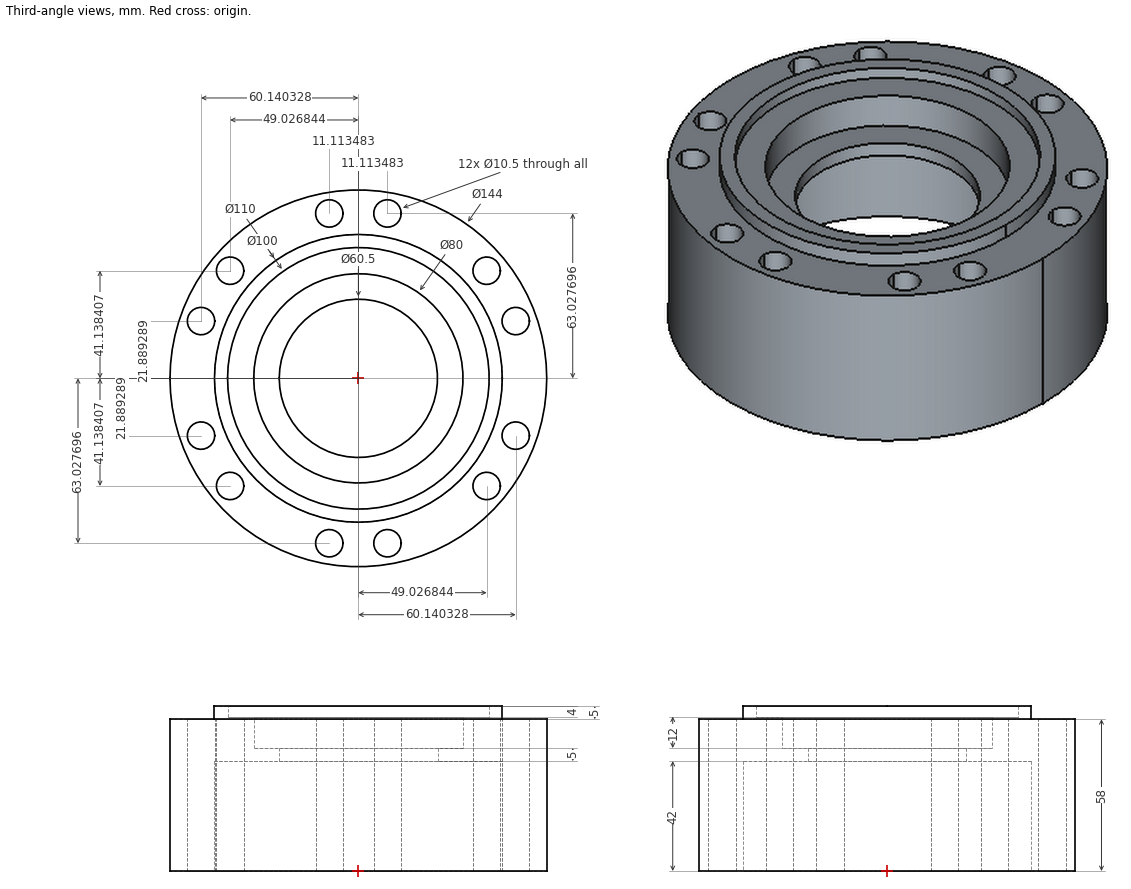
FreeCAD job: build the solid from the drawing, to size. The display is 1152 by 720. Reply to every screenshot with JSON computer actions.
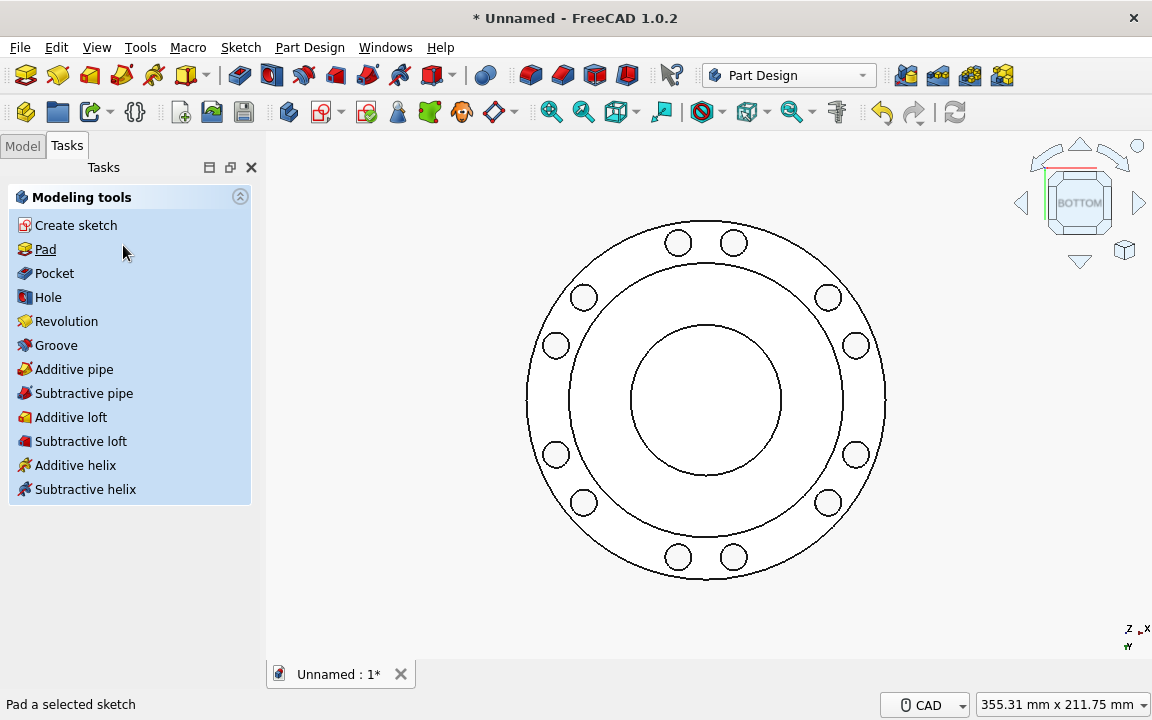
{"action": "left_click", "coordinate": [240, 76]}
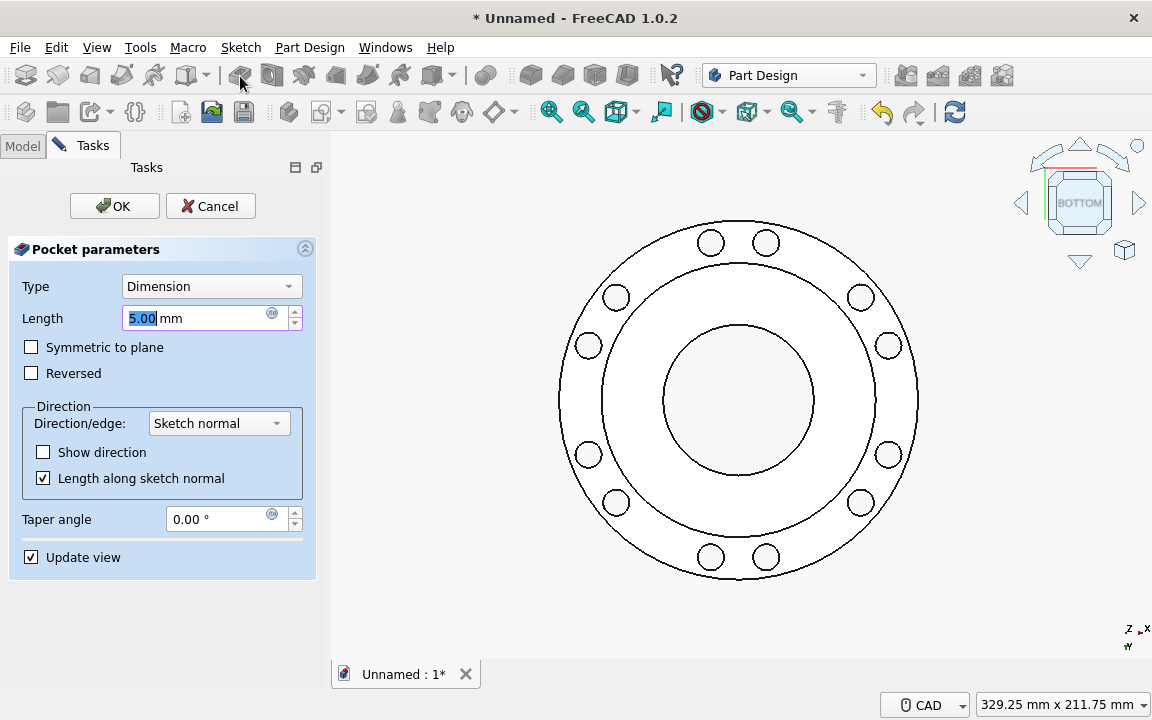
{"action": "type", "text": "4"}
{"action": "key", "text": "Tab"}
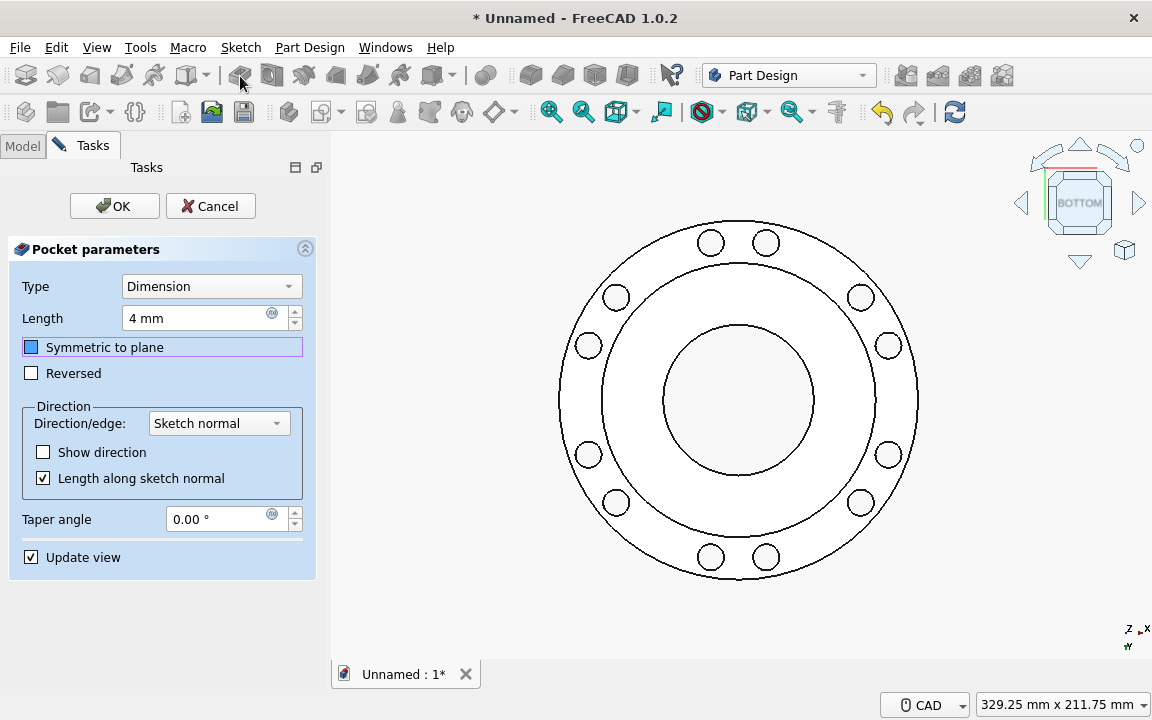
{"action": "left_click", "coordinate": [115, 206]}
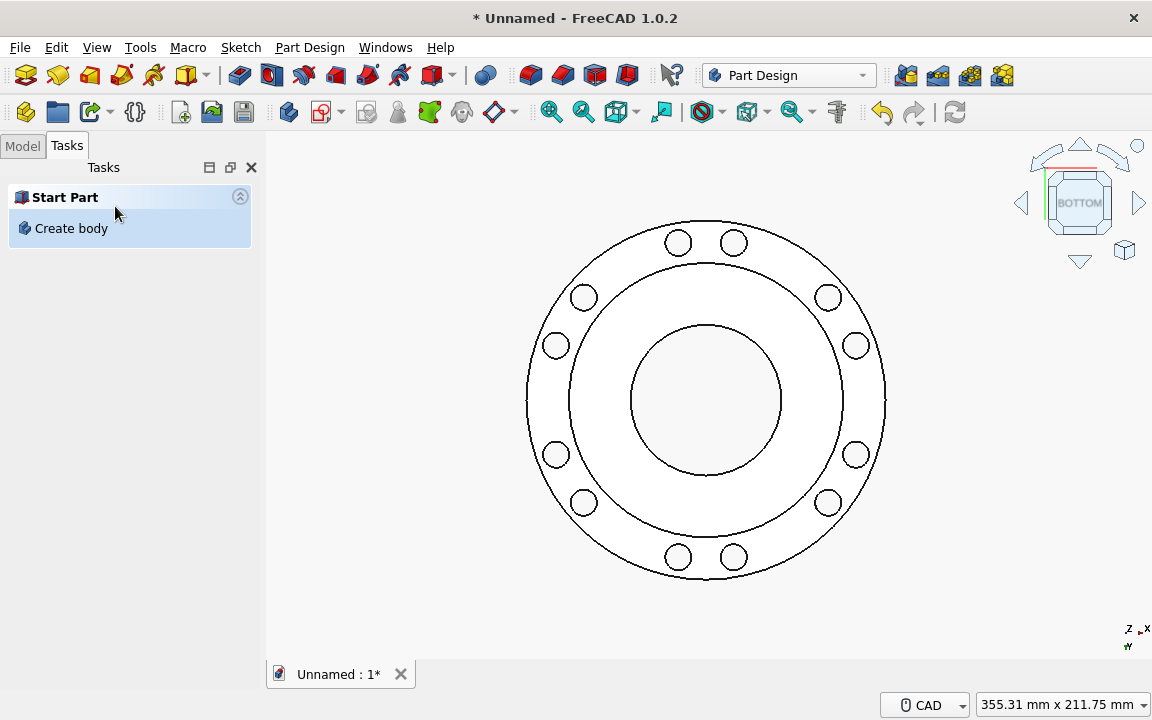
{"action": "key", "text": "0"}